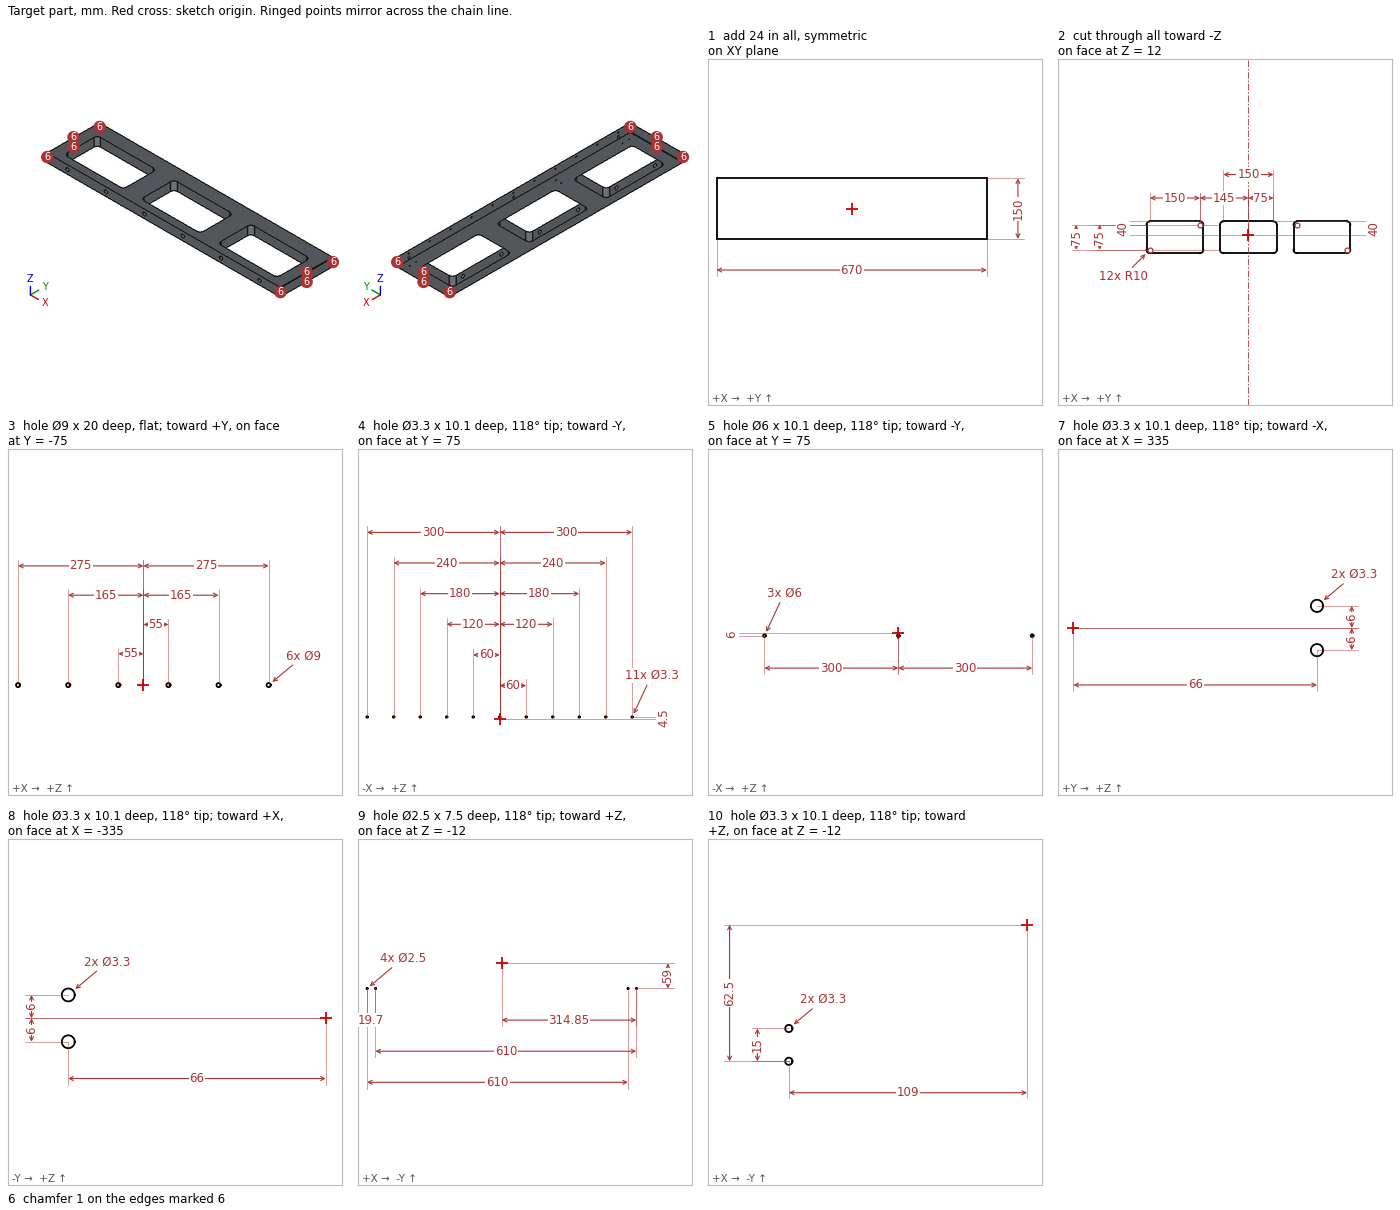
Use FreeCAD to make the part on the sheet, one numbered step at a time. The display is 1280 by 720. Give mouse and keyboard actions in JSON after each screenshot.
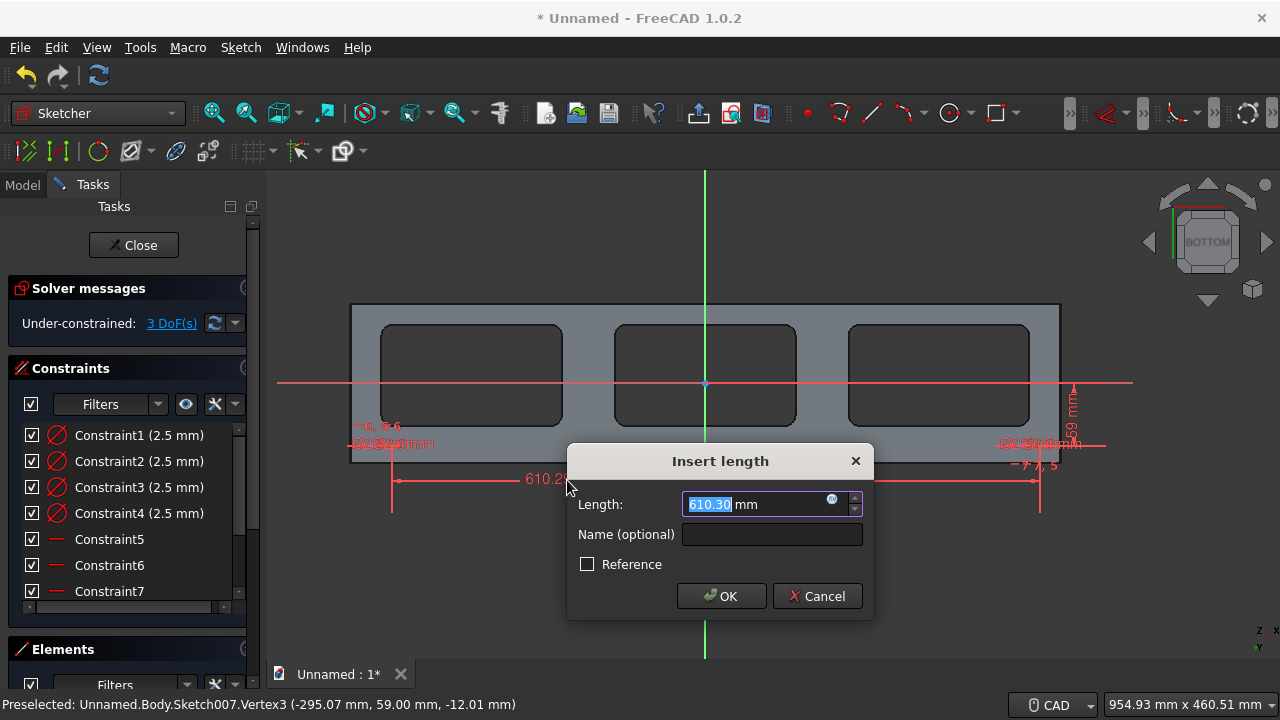
{"action": "type", "text": "610"}
{"action": "key", "text": "Return"}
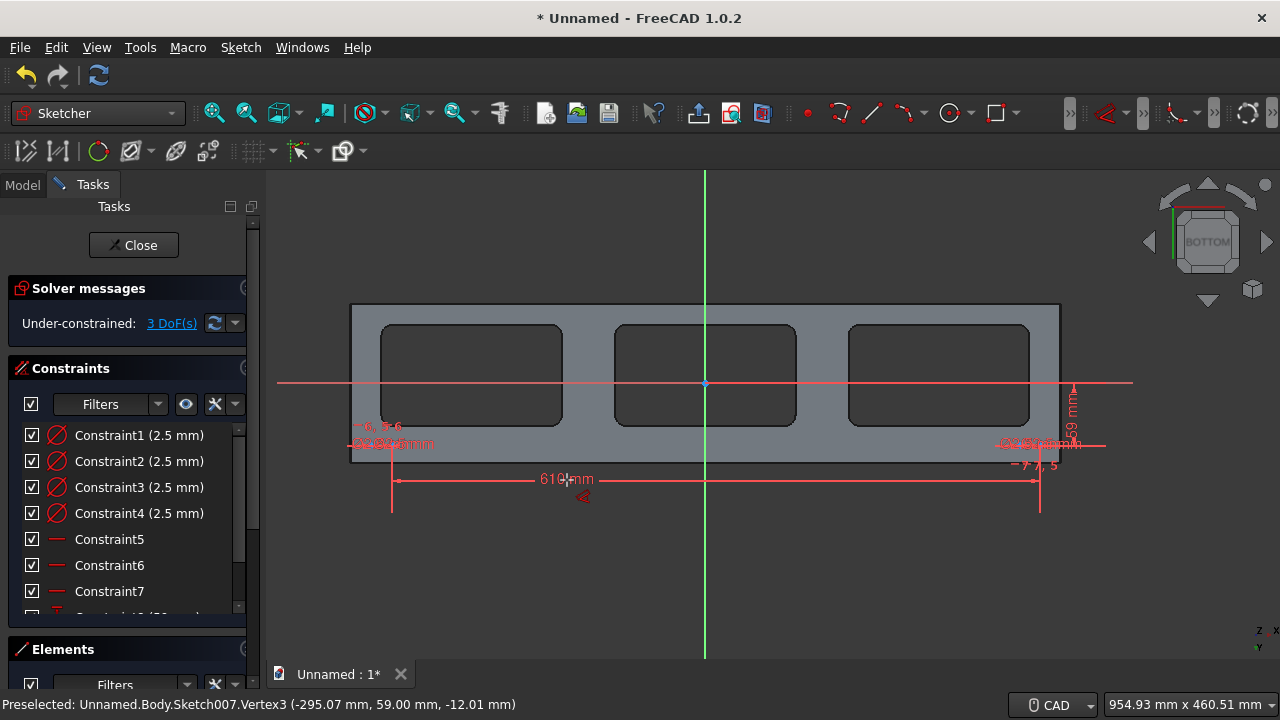
{"action": "left_click", "coordinate": [371, 446]}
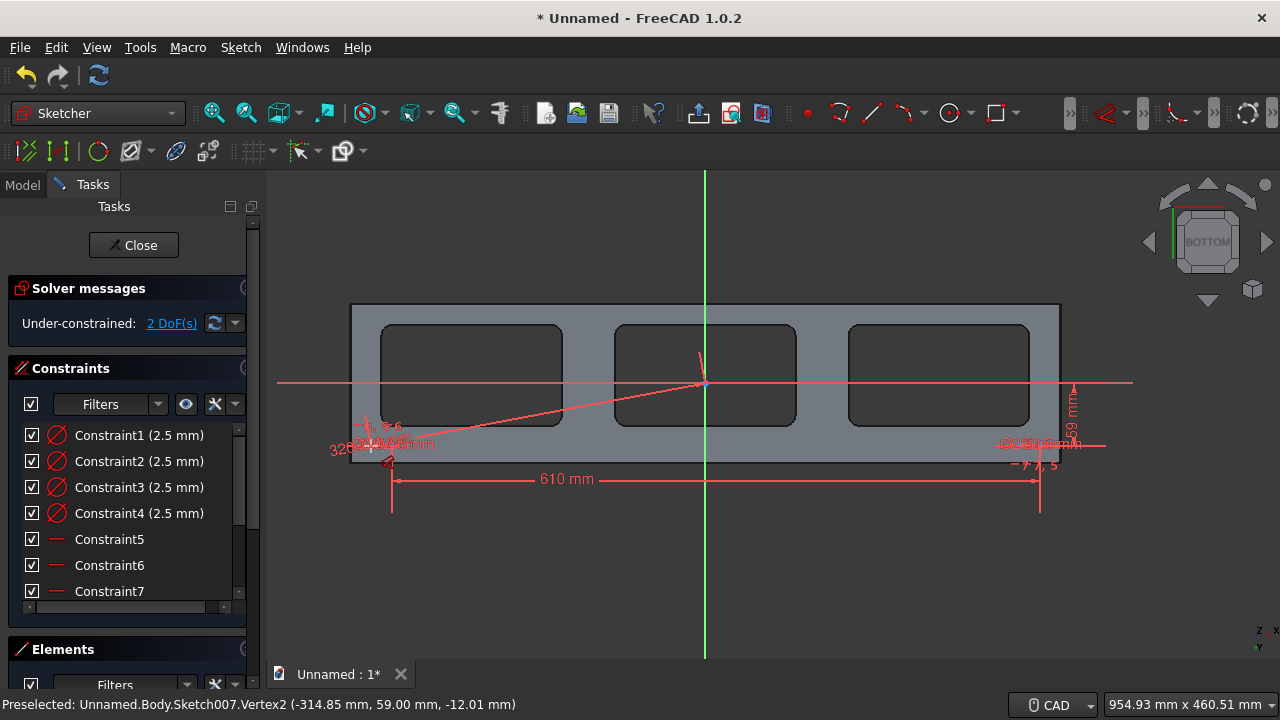
{"action": "left_click", "coordinate": [1019, 446]}
{"action": "left_click", "coordinate": [844, 480]}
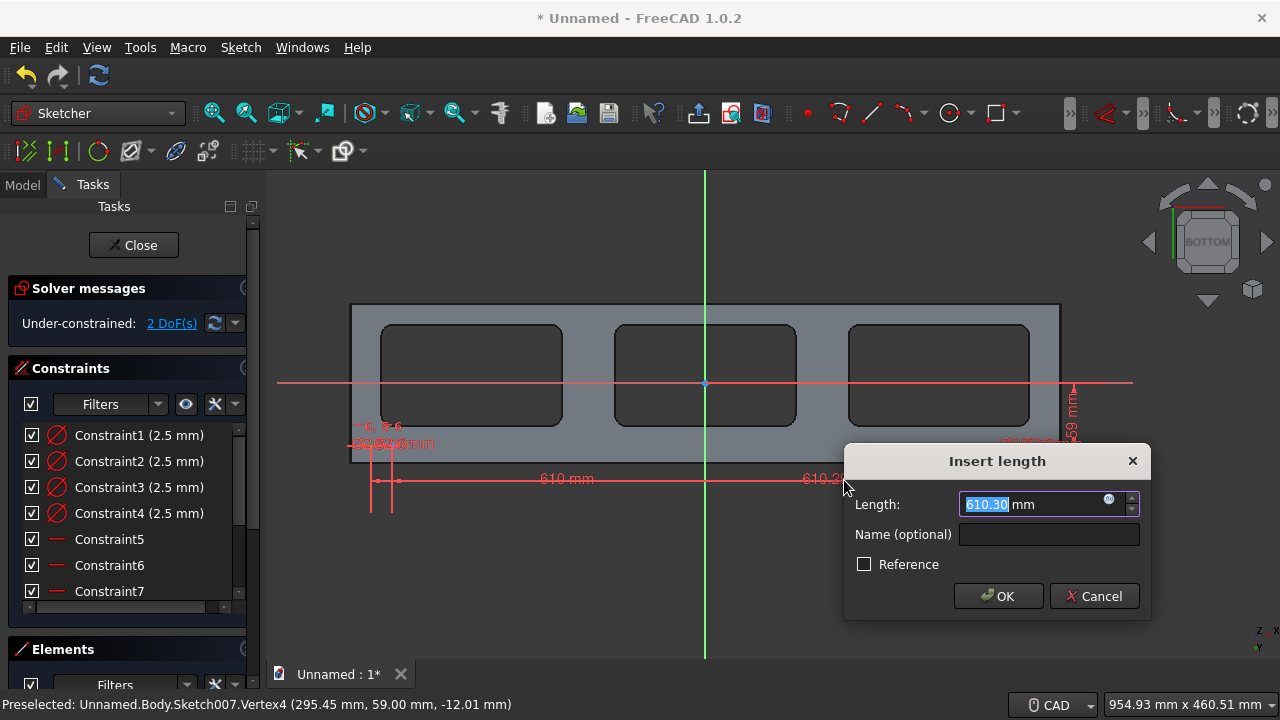
{"action": "type", "text": "610"}
{"action": "key", "text": "Return"}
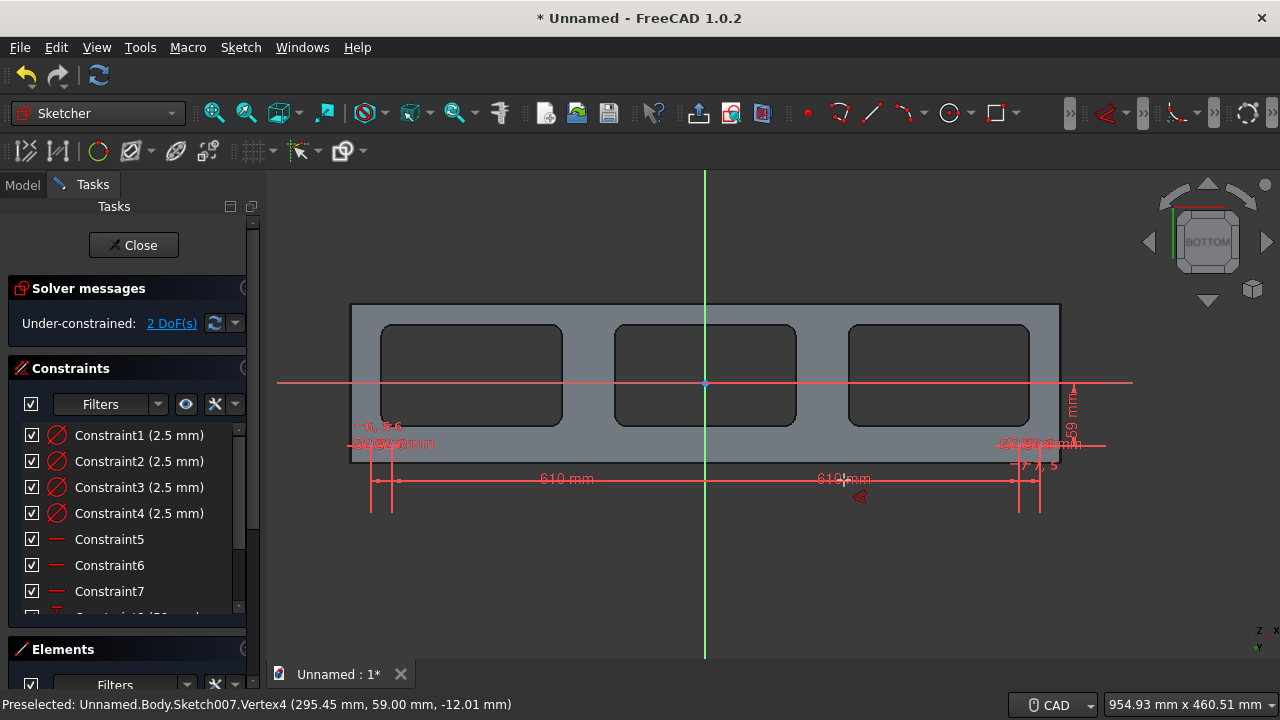
{"action": "scroll", "coordinate": [371, 446], "scroll_direction": "up", "scroll_amount": 4}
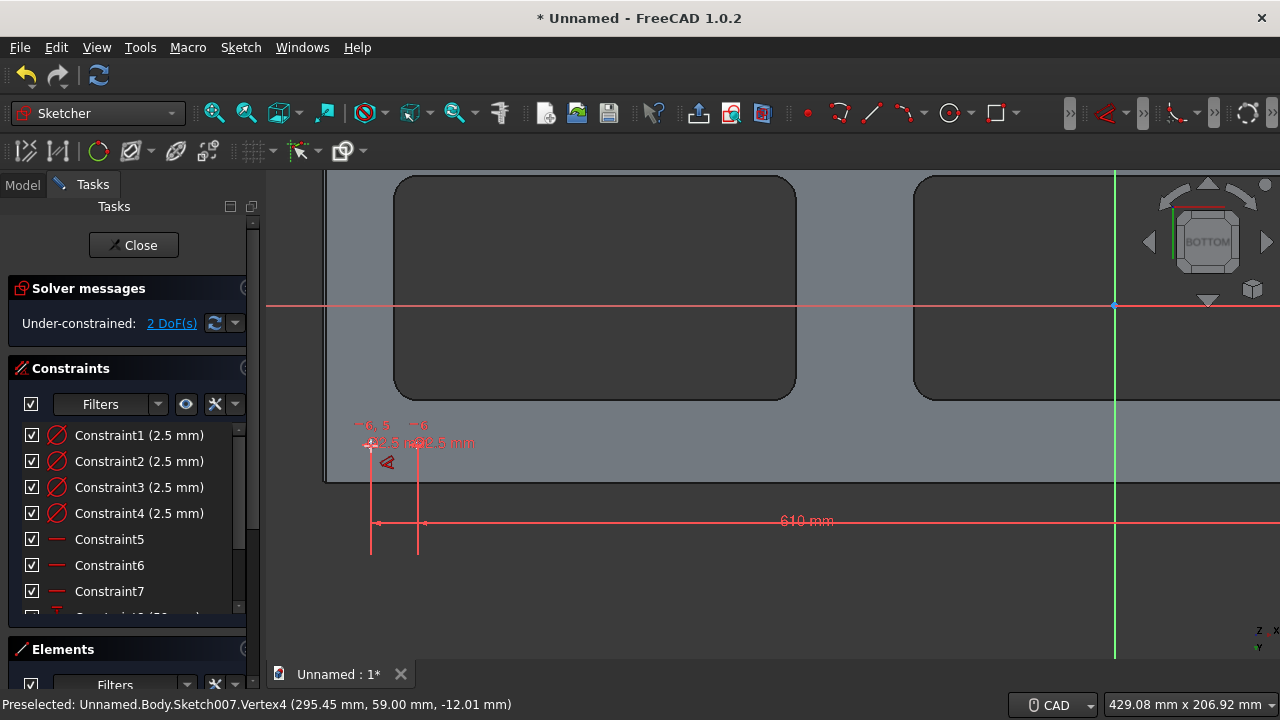
{"action": "left_click", "coordinate": [371, 445]}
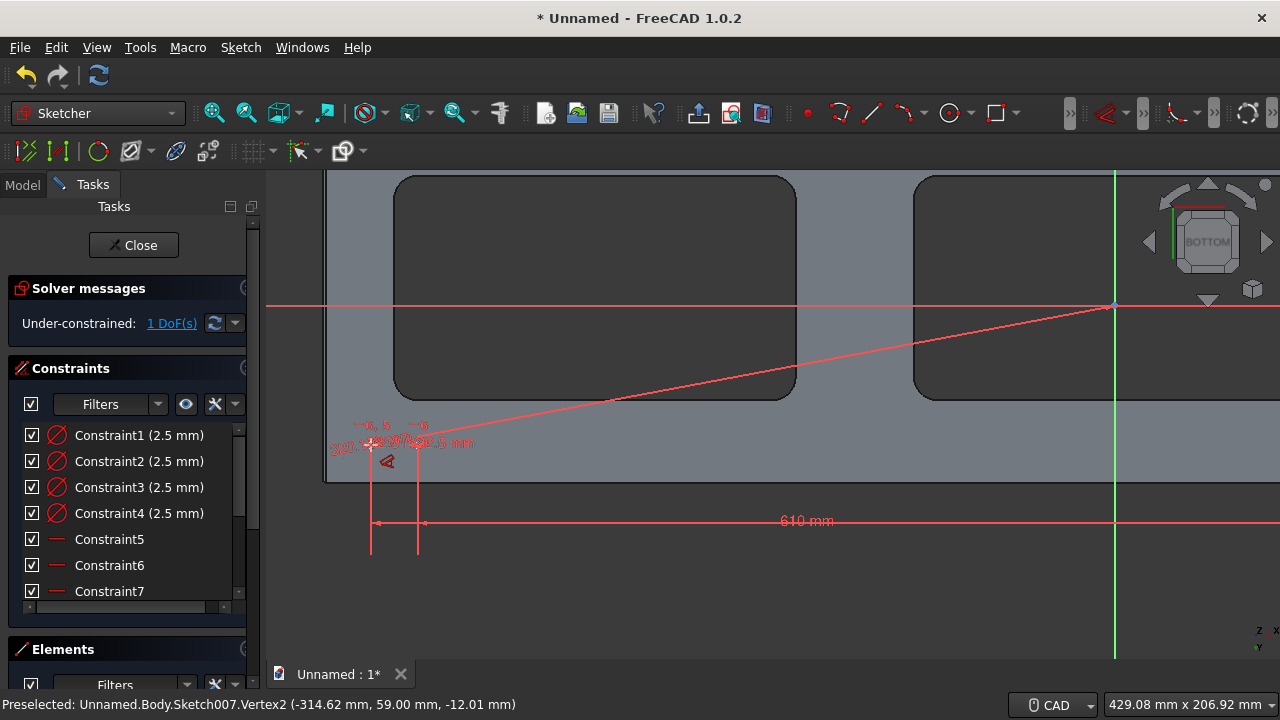
{"action": "left_click", "coordinate": [418, 445]}
{"action": "left_click", "coordinate": [395, 479]}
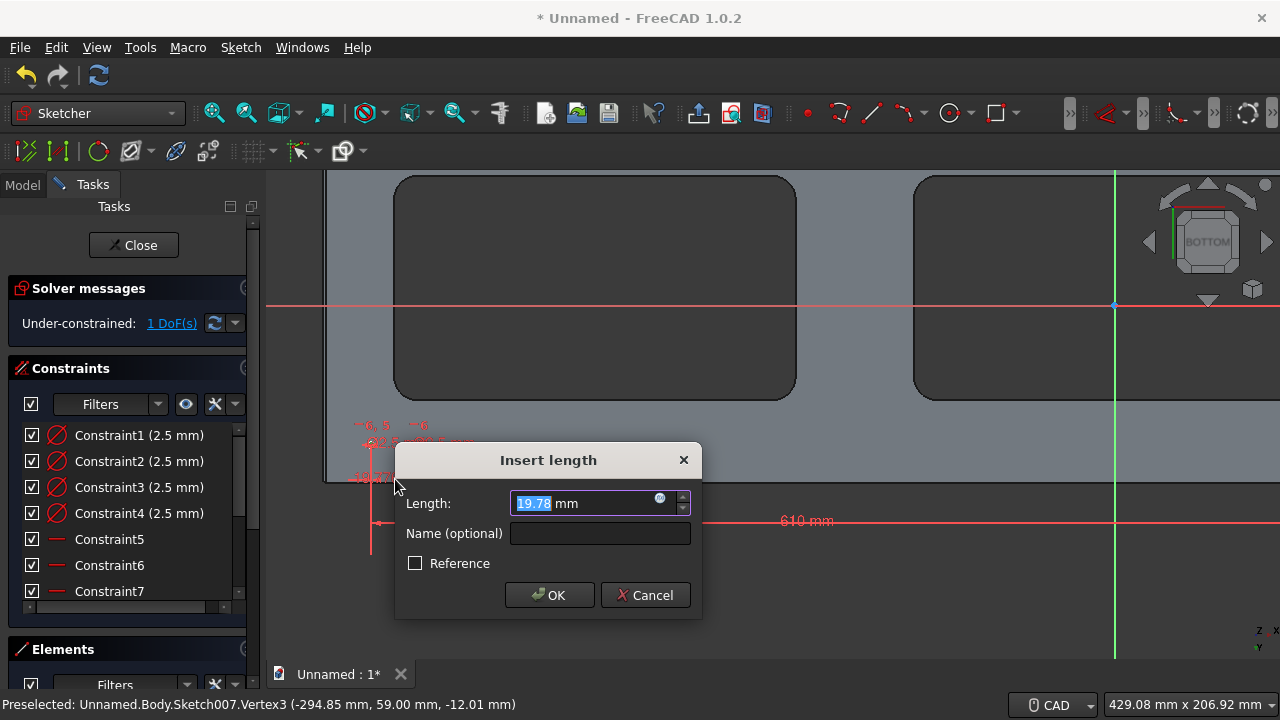
{"action": "type", "text": "19.7"}
{"action": "key", "text": "Return"}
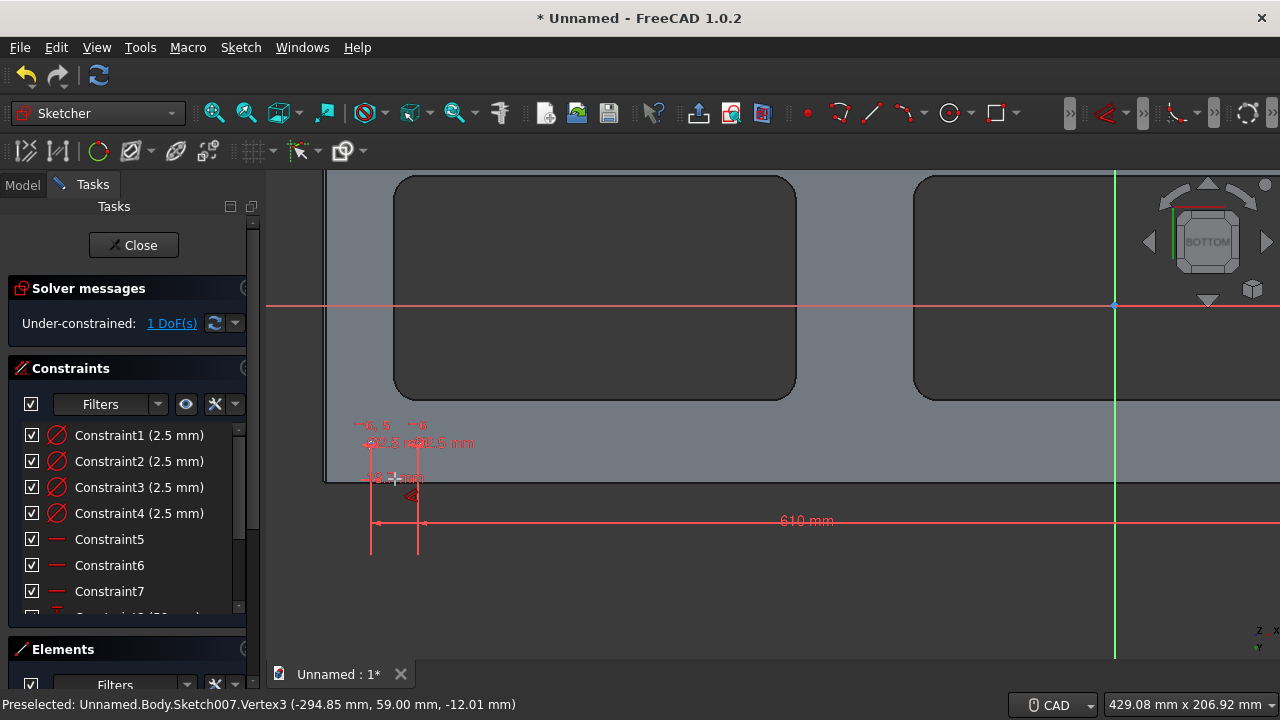
{"action": "scroll", "coordinate": [466, 436], "scroll_direction": "down", "scroll_amount": 5}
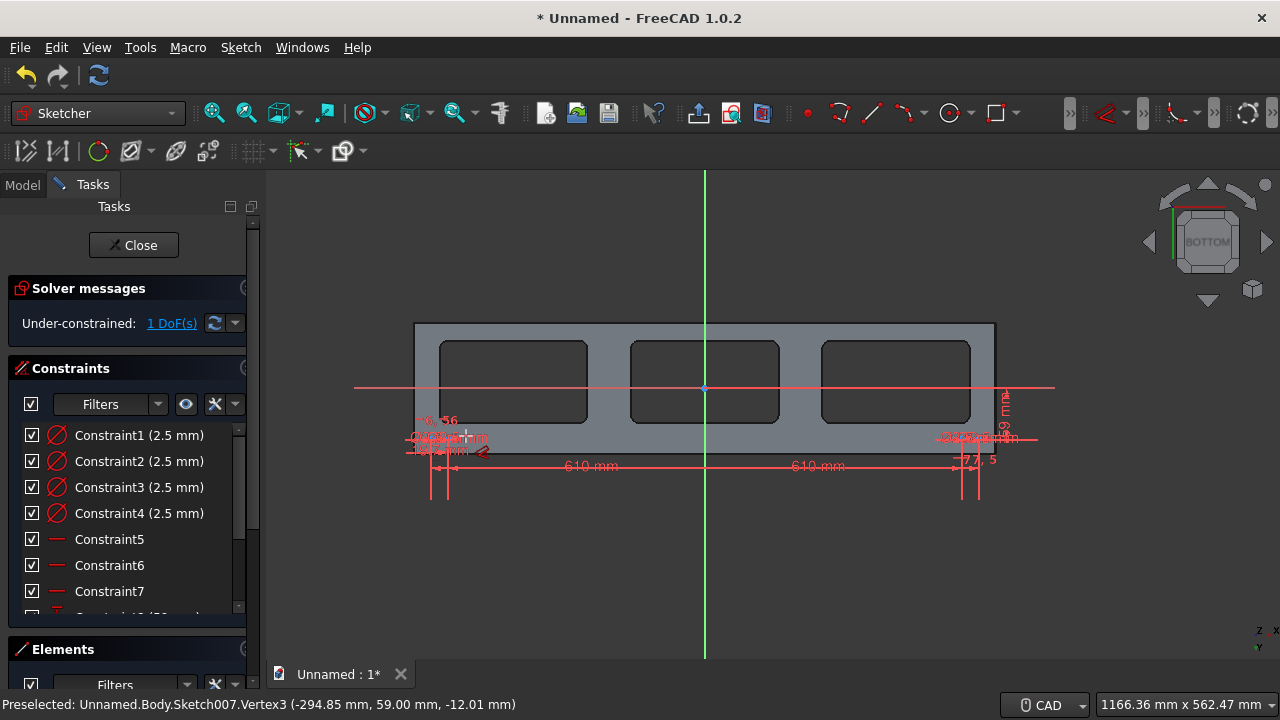
{"action": "left_click", "coordinate": [979, 440]}
{"action": "left_click", "coordinate": [842, 354]}